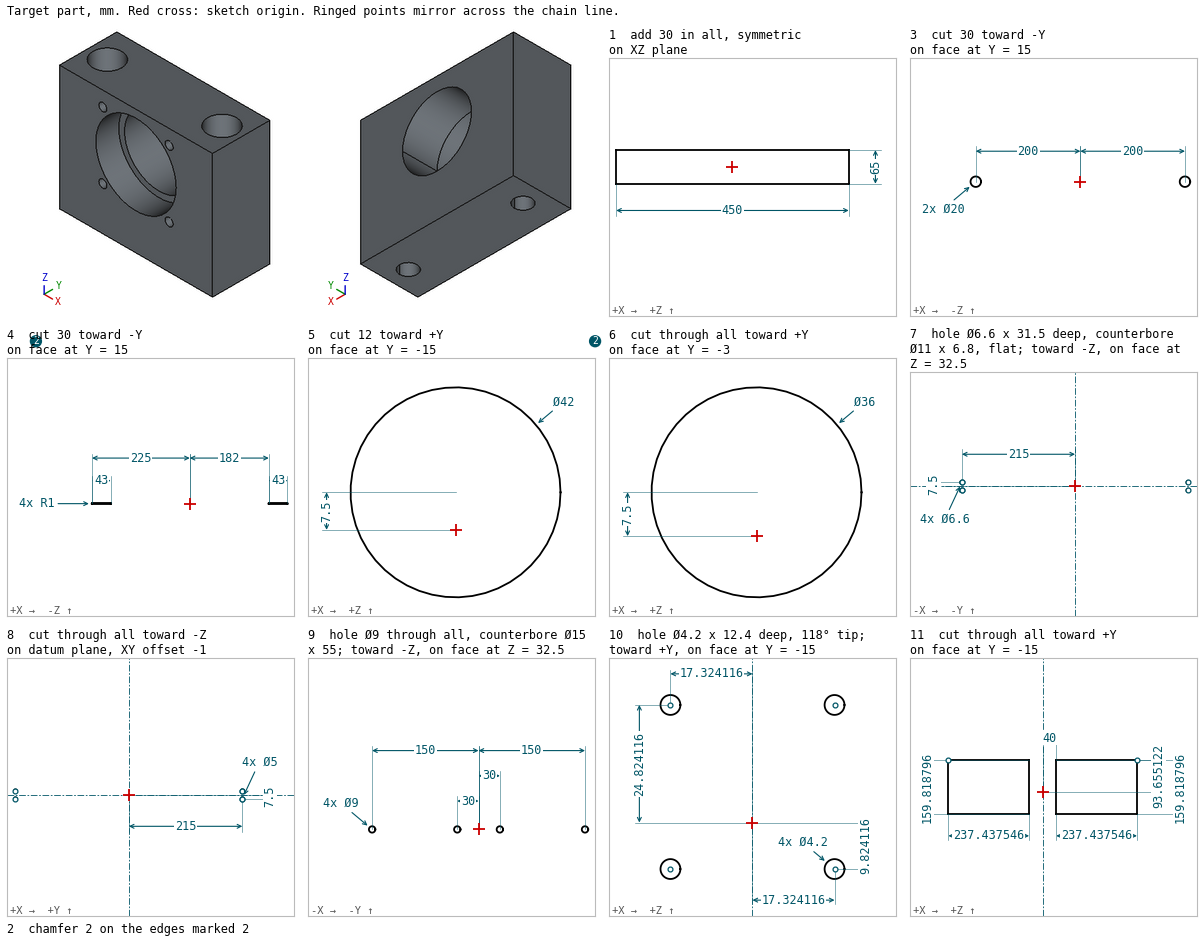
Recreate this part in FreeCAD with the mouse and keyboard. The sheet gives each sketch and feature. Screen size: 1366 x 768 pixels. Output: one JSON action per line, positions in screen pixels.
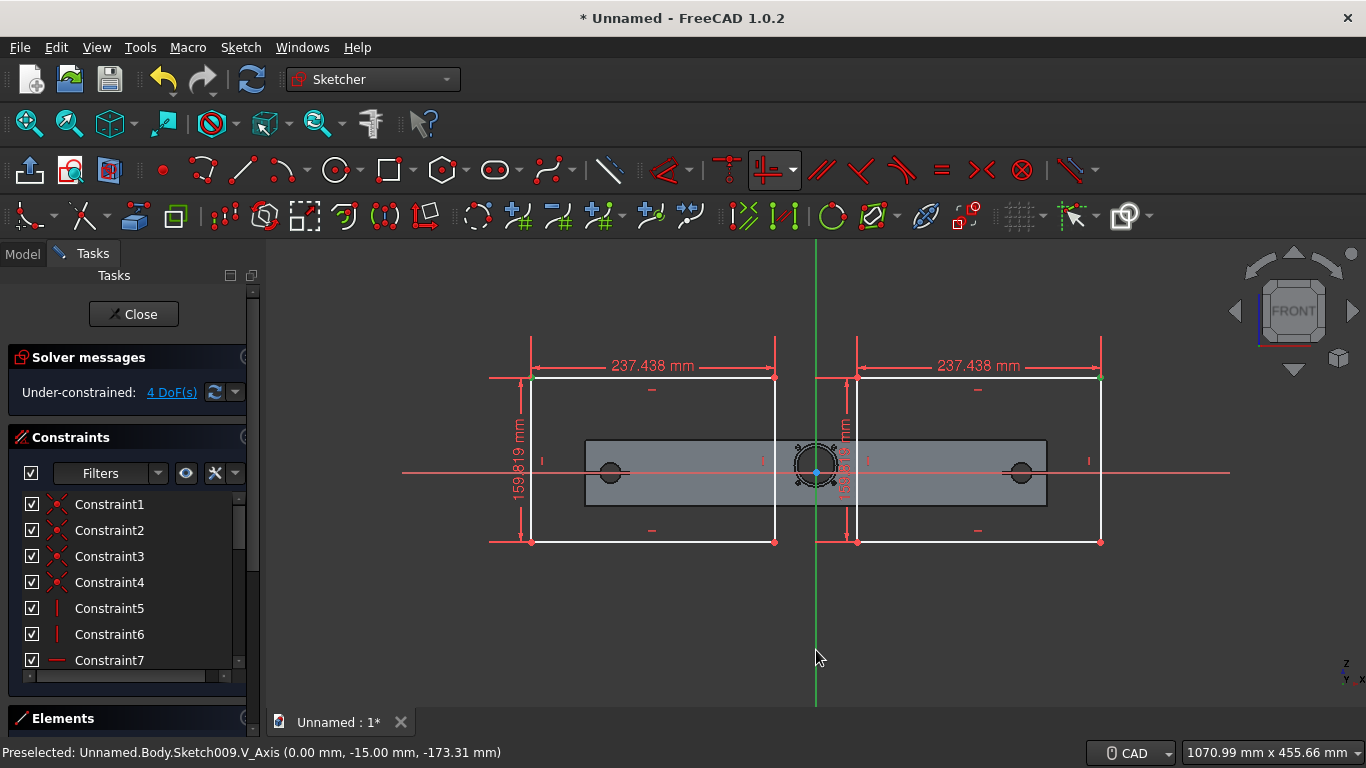
{"action": "key", "text": "s"}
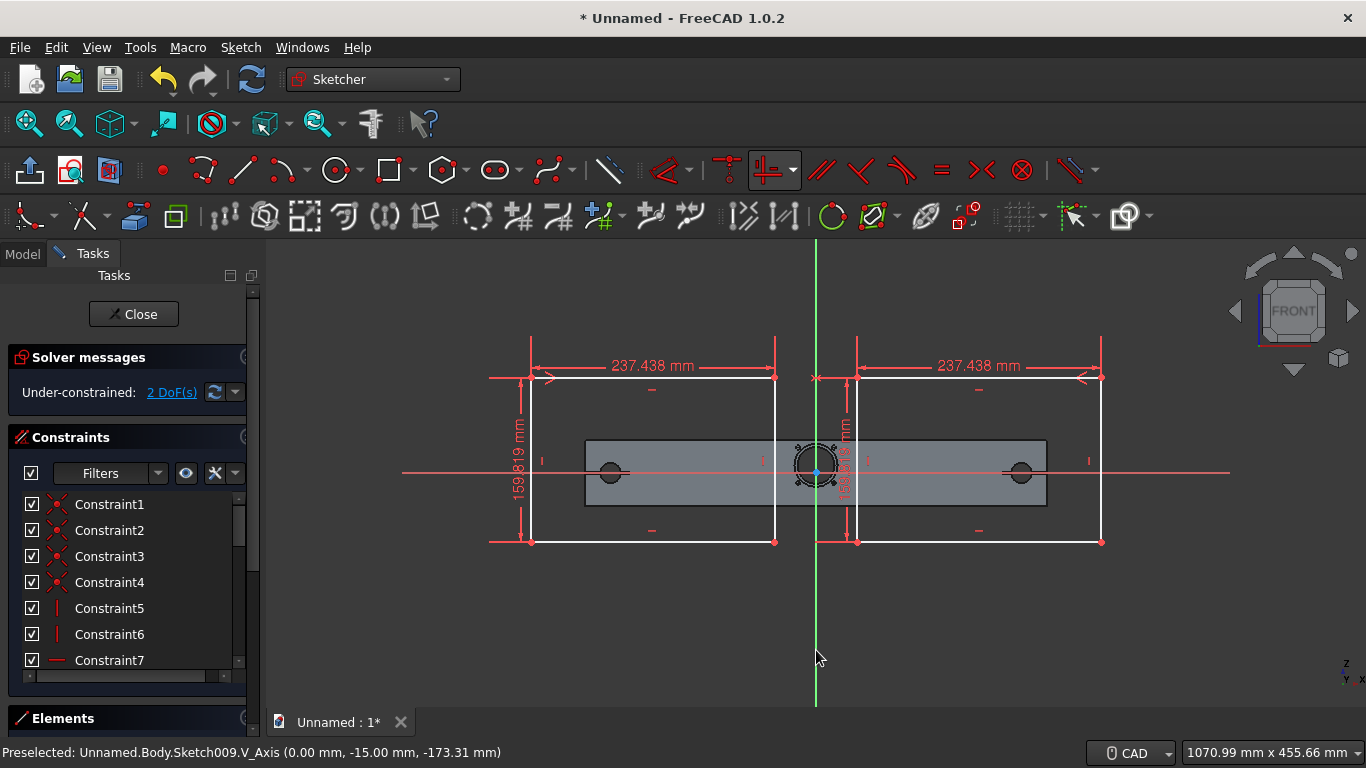
{"action": "left_click", "coordinate": [664, 170]}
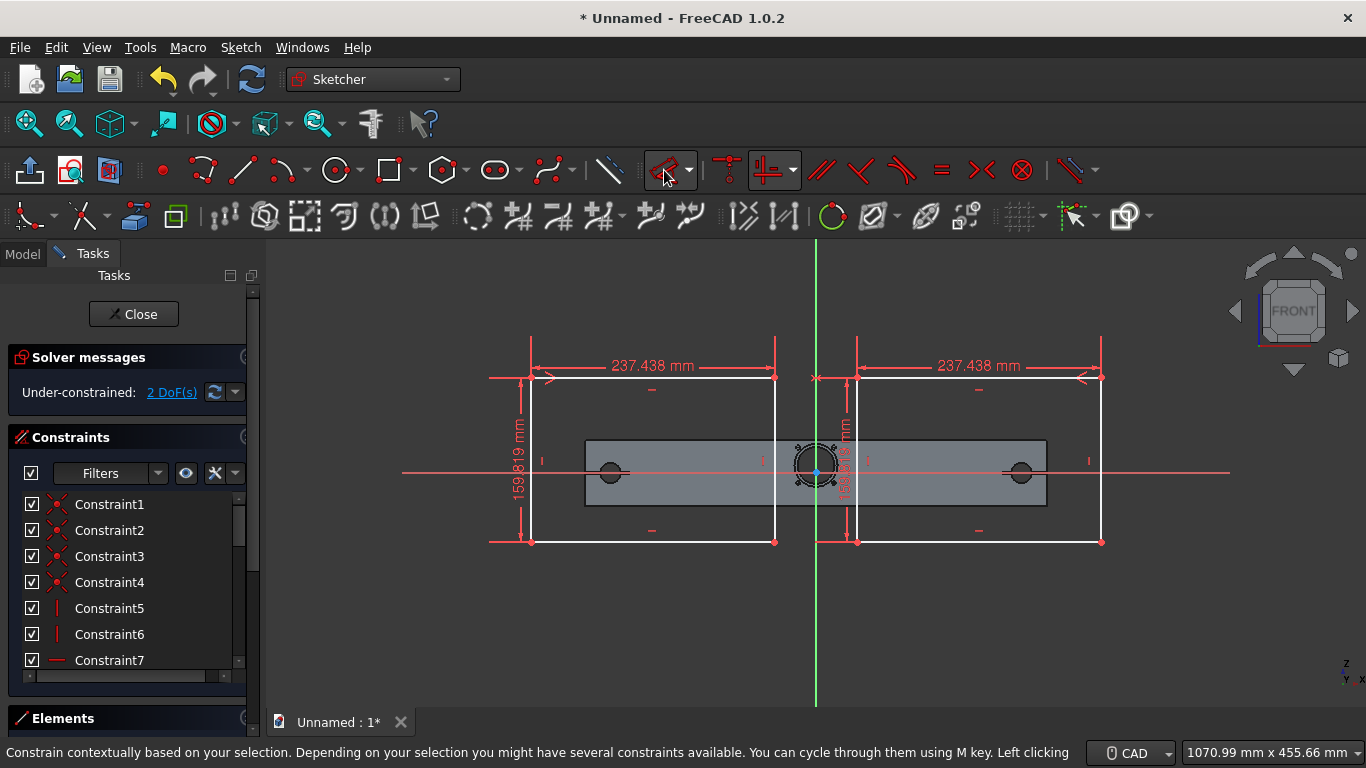
{"action": "left_click", "coordinate": [857, 378]}
{"action": "left_click", "coordinate": [837, 344]}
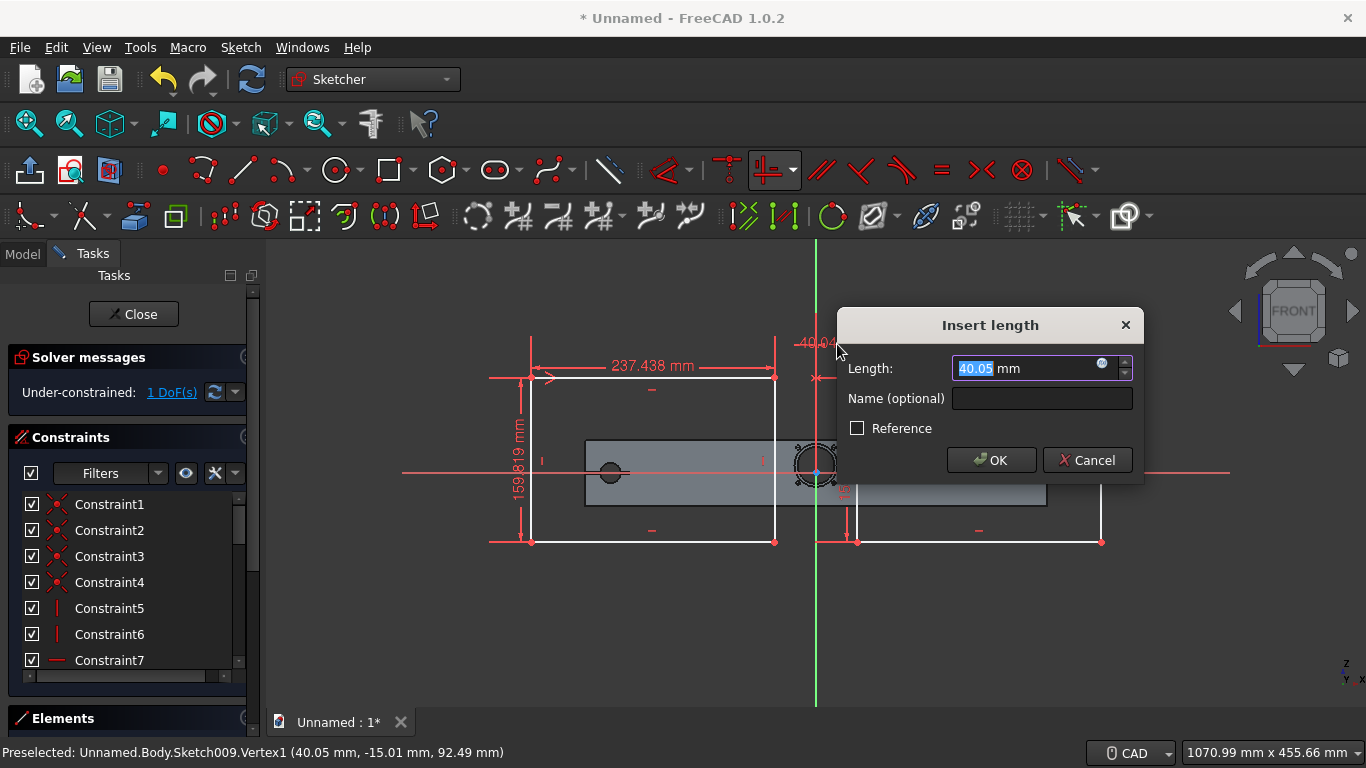
{"action": "type", "text": "40"}
{"action": "key", "text": "Return"}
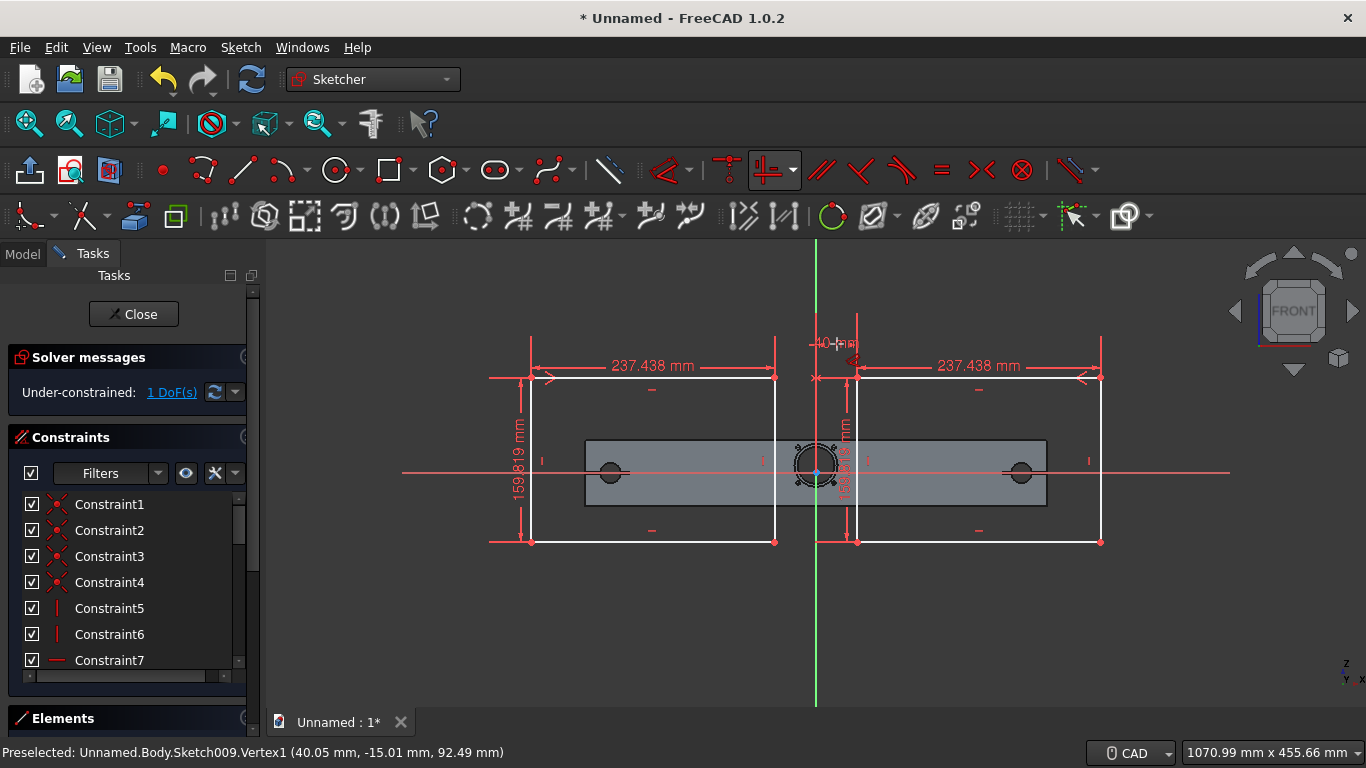
{"action": "left_click", "coordinate": [857, 378]}
{"action": "left_click", "coordinate": [891, 426]}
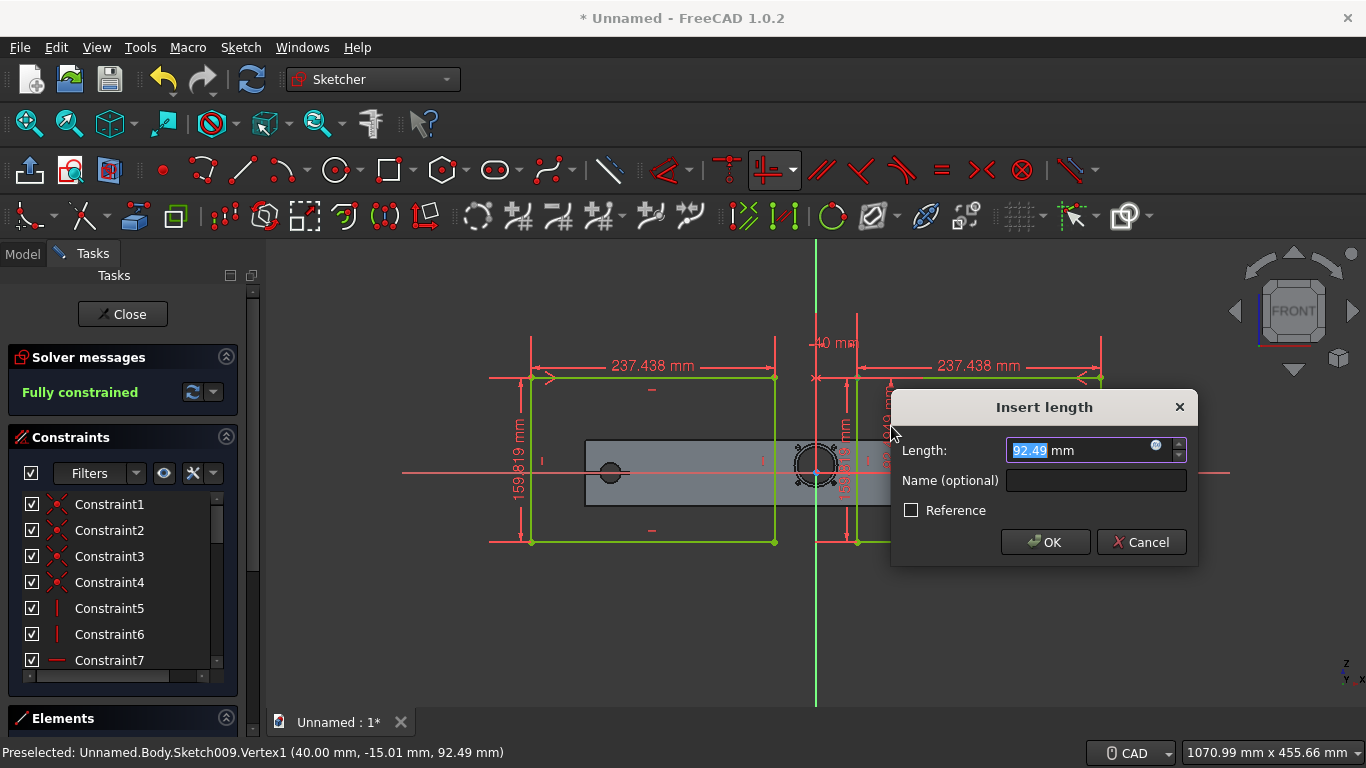
{"action": "type", "text": "93.655122"}
{"action": "key", "text": "Return"}
{"action": "key", "text": "Escape"}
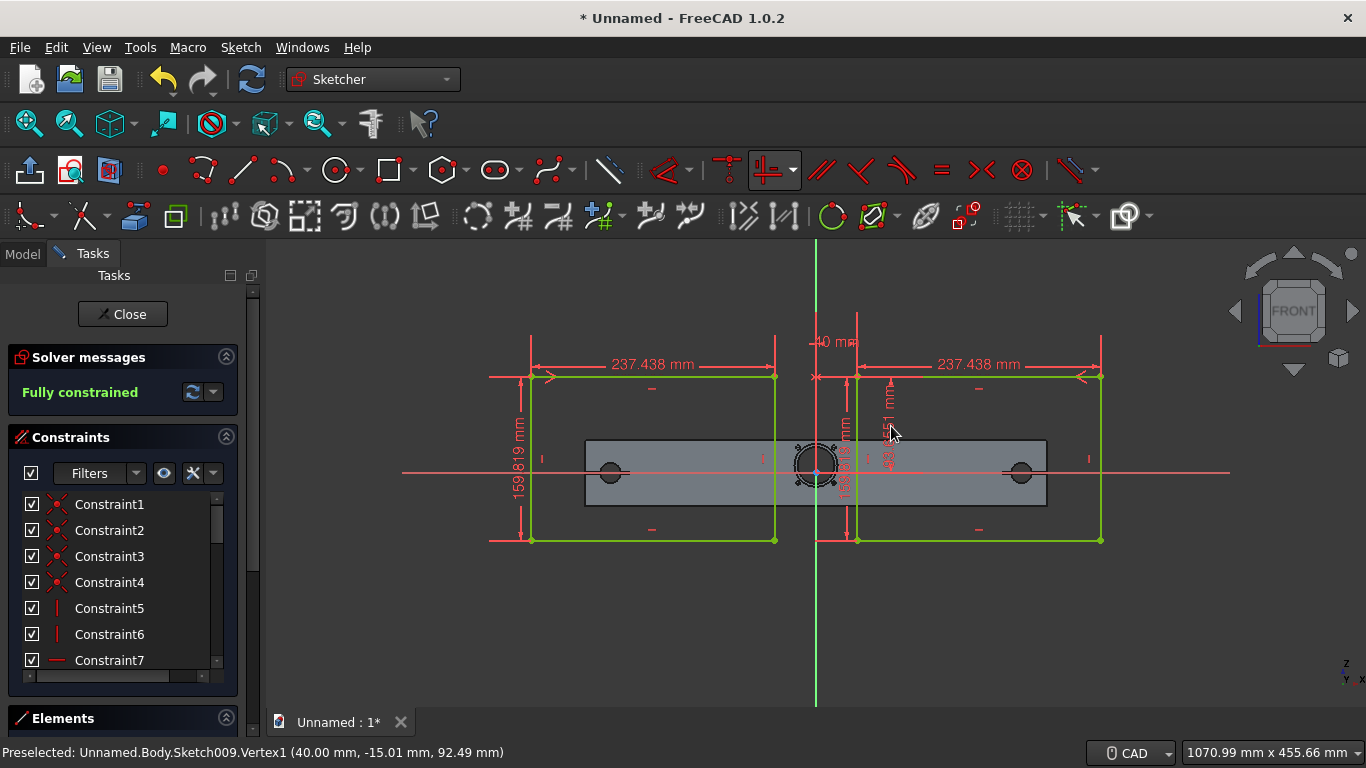
{"action": "left_click", "coordinate": [123, 314]}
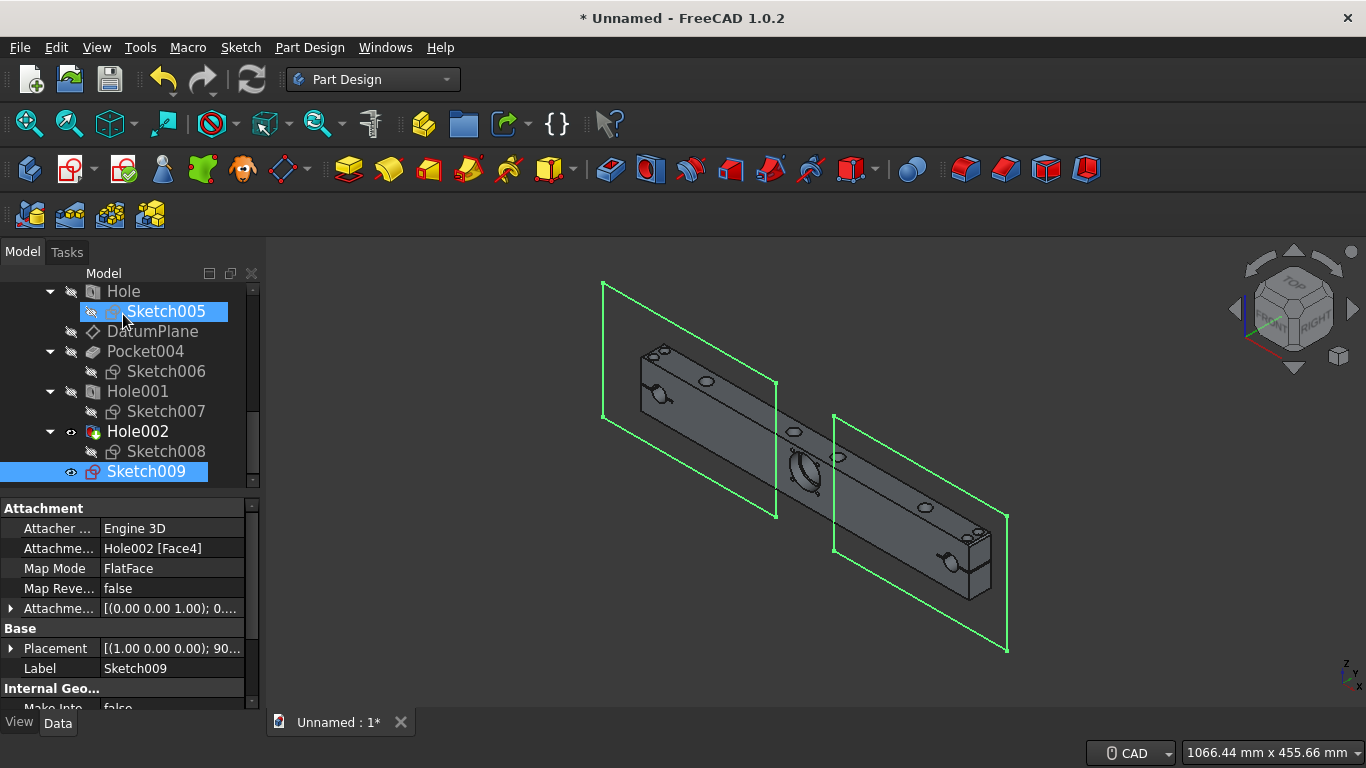
{"action": "left_click", "coordinate": [612, 170]}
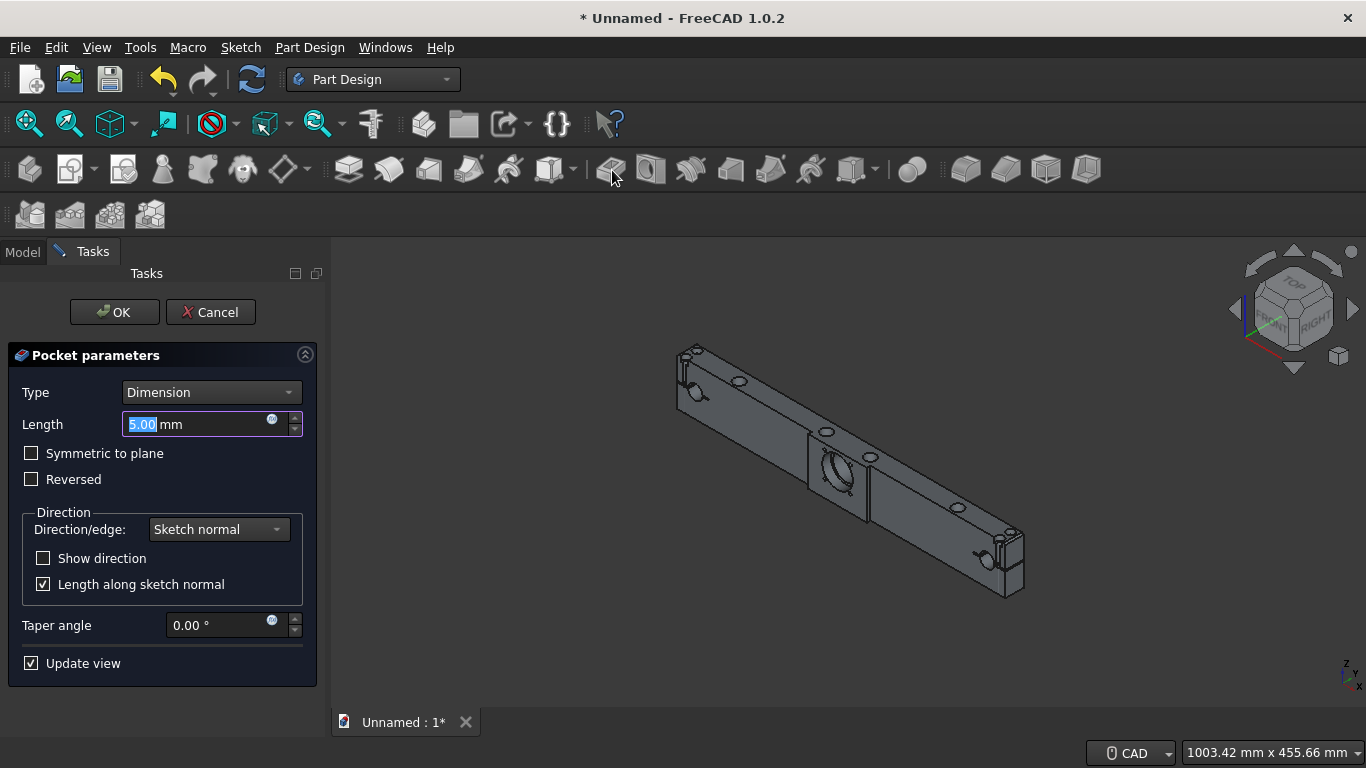
{"action": "left_click", "coordinate": [212, 392]}